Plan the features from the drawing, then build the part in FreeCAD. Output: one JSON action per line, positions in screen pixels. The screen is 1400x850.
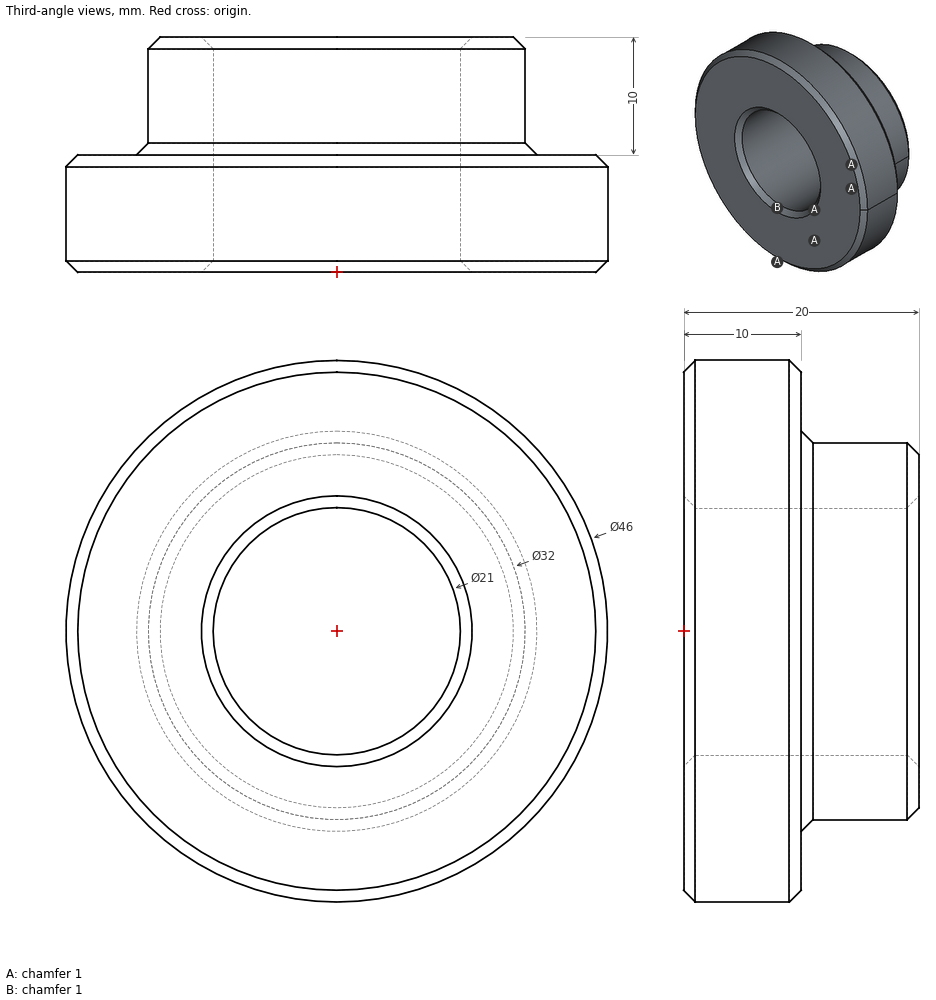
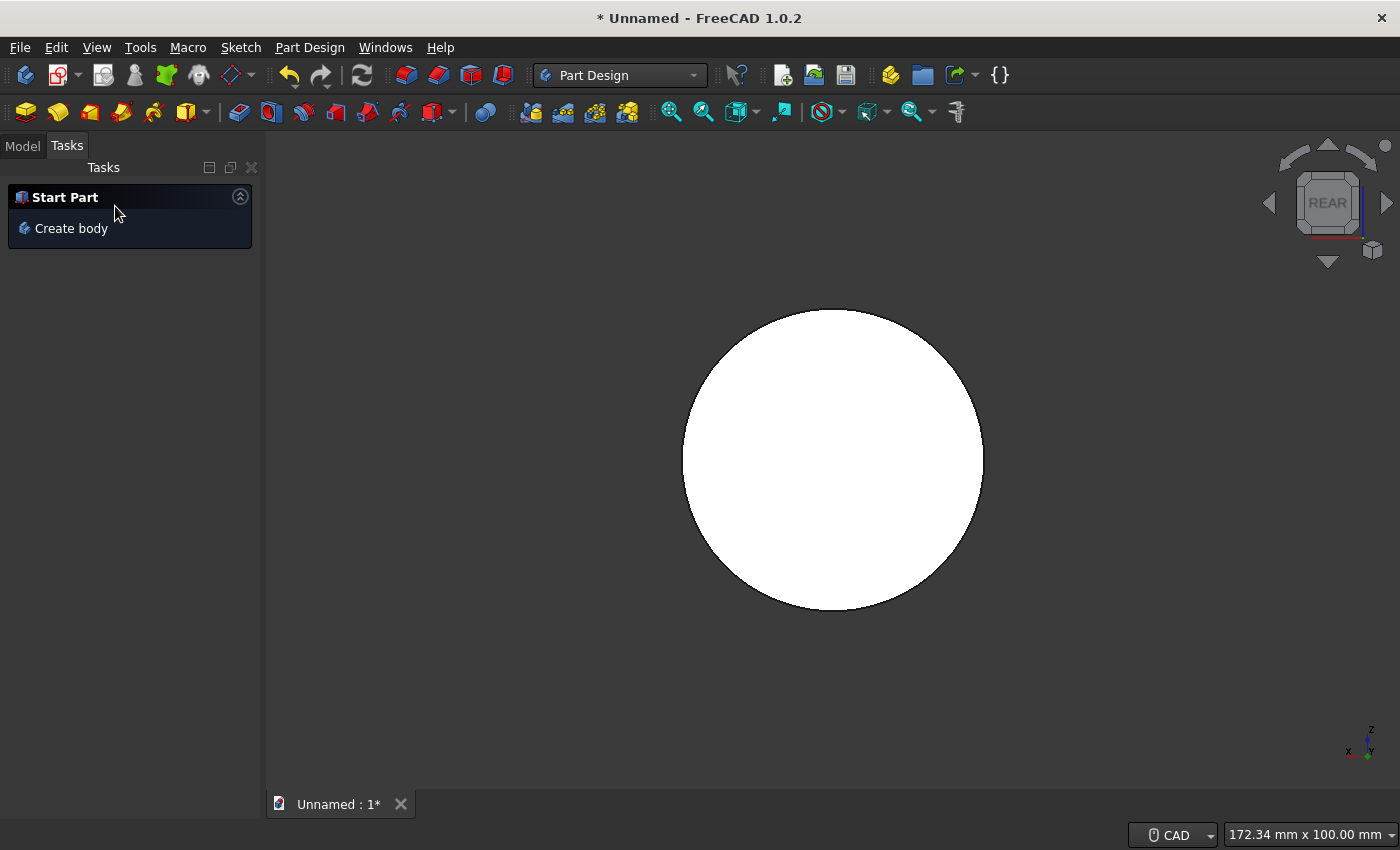
{"action": "left_click", "coordinate": [833, 459]}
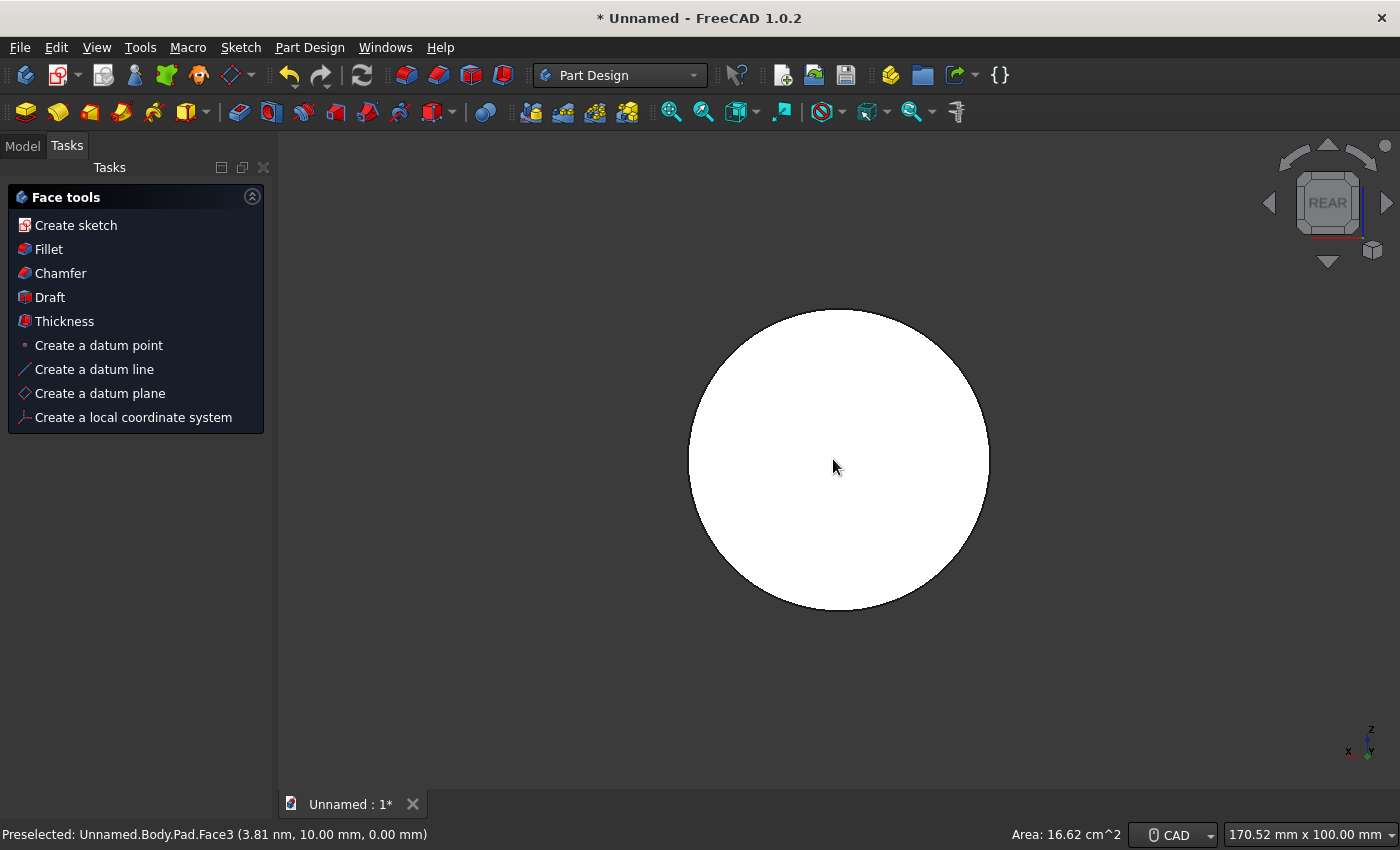
{"action": "left_click", "coordinate": [58, 76]}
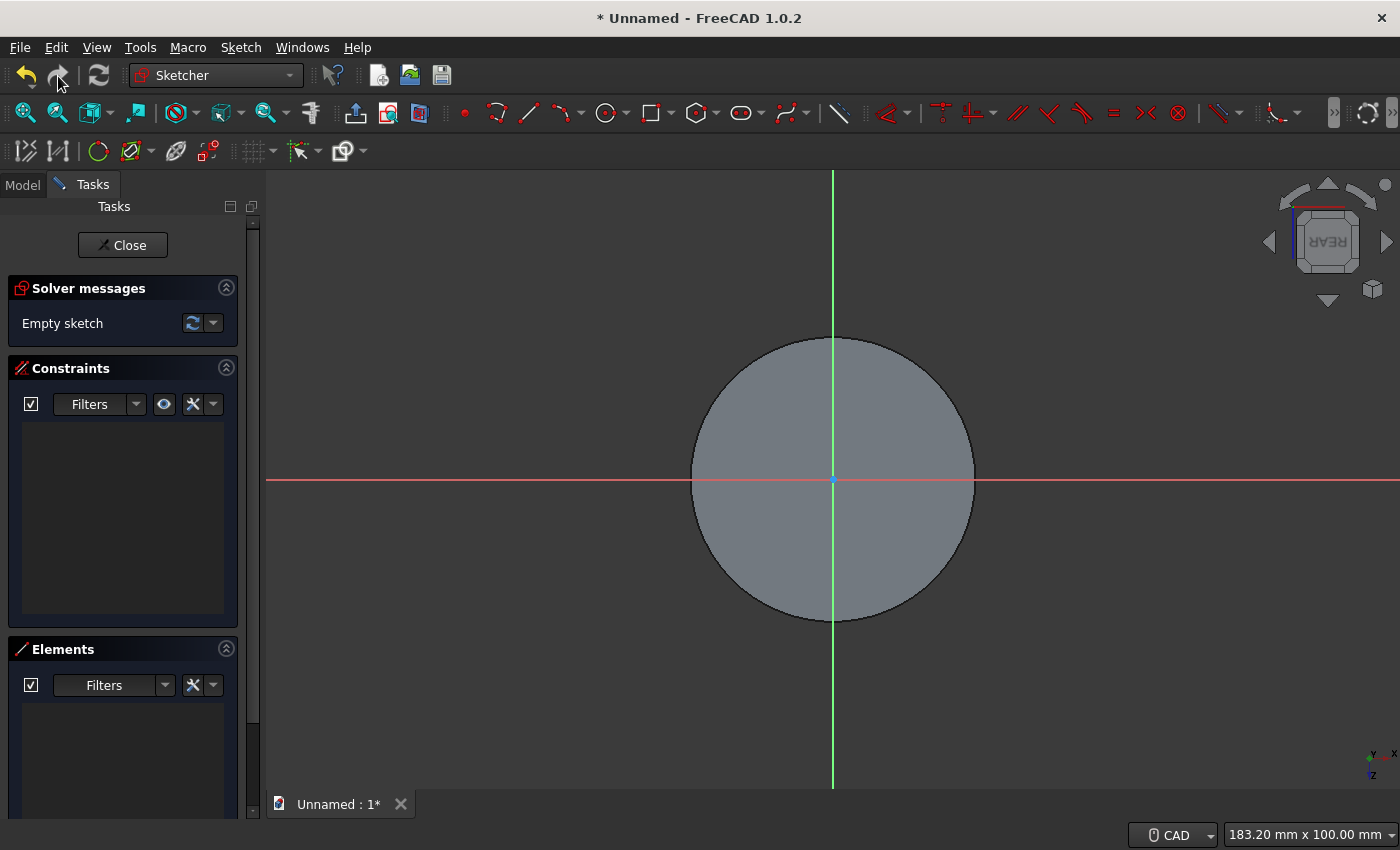
{"action": "scroll", "coordinate": [916, 480], "scroll_direction": "up", "scroll_amount": 3}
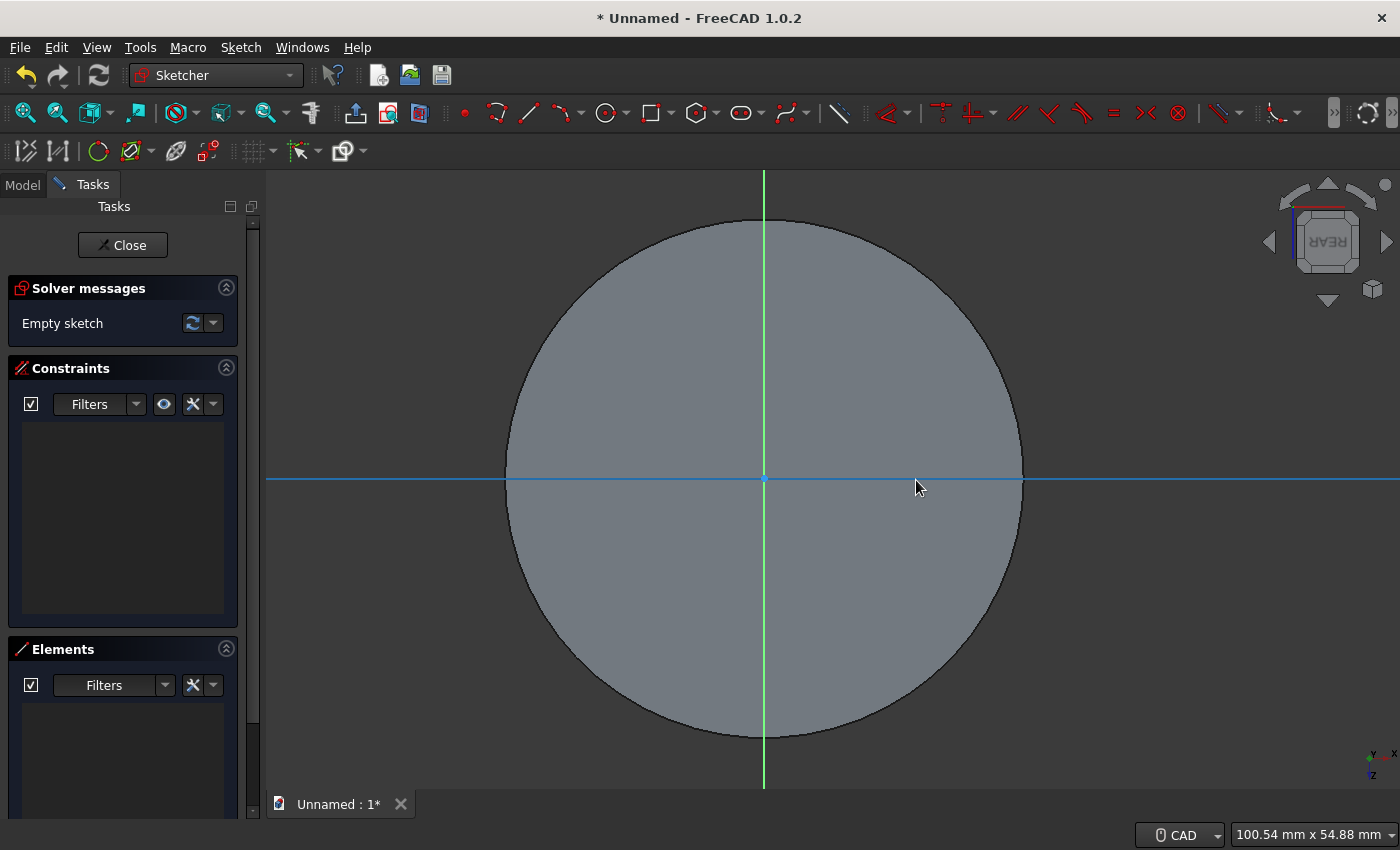
{"action": "key", "text": "g c"}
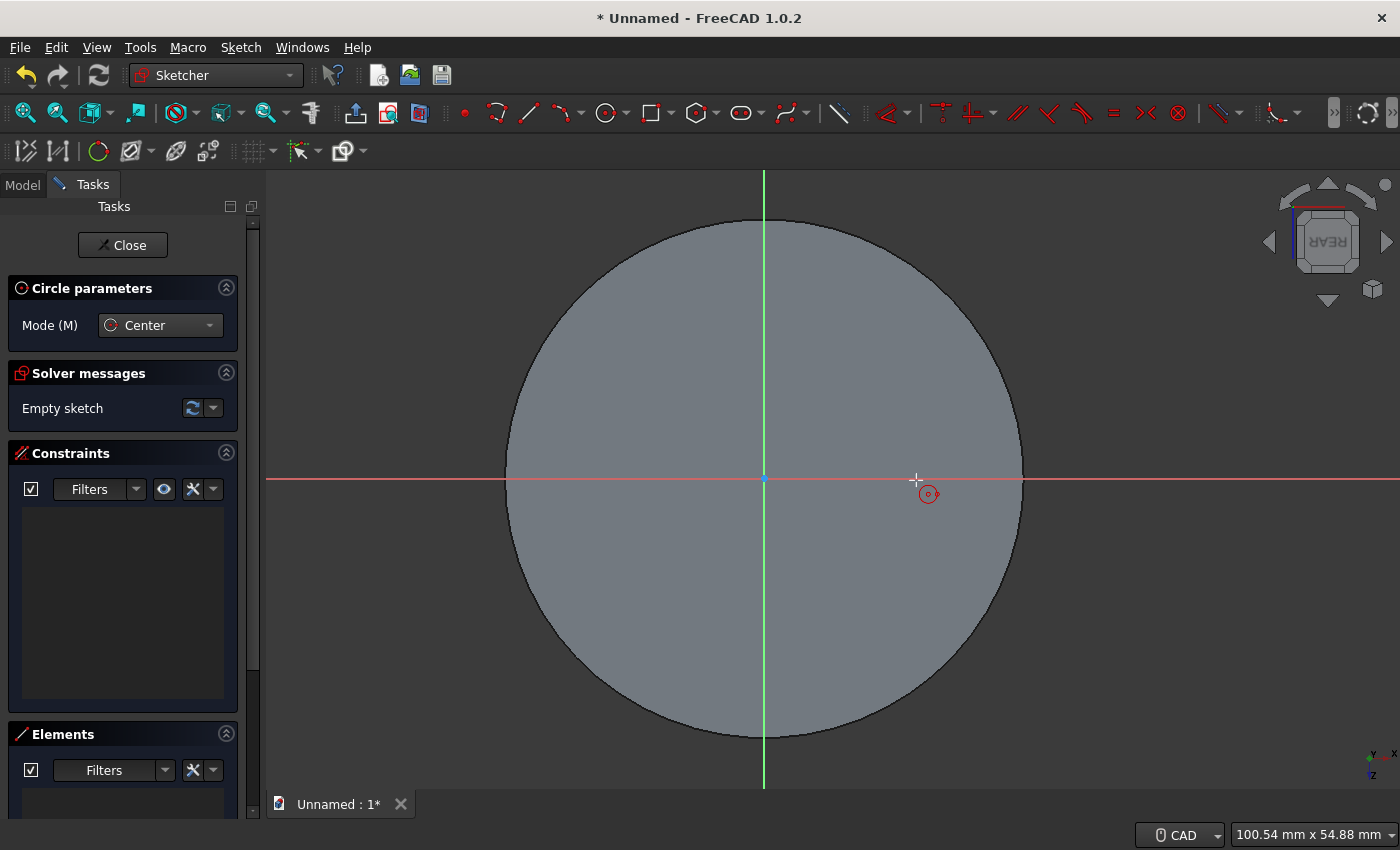
{"action": "left_click", "coordinate": [764, 479]}
{"action": "left_click", "coordinate": [892, 351]}
{"action": "key", "text": "Escape"}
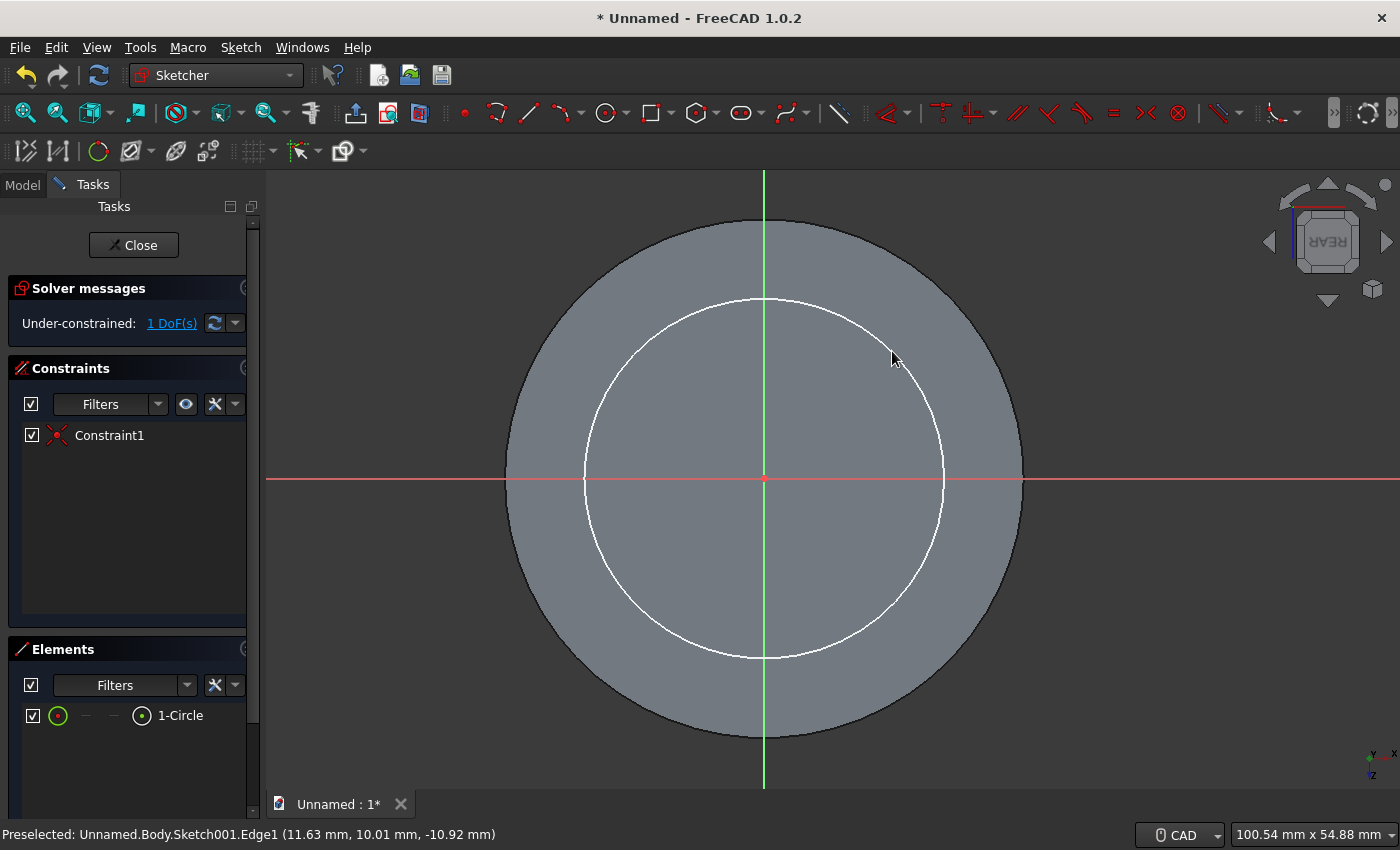
{"action": "left_click", "coordinate": [886, 114]}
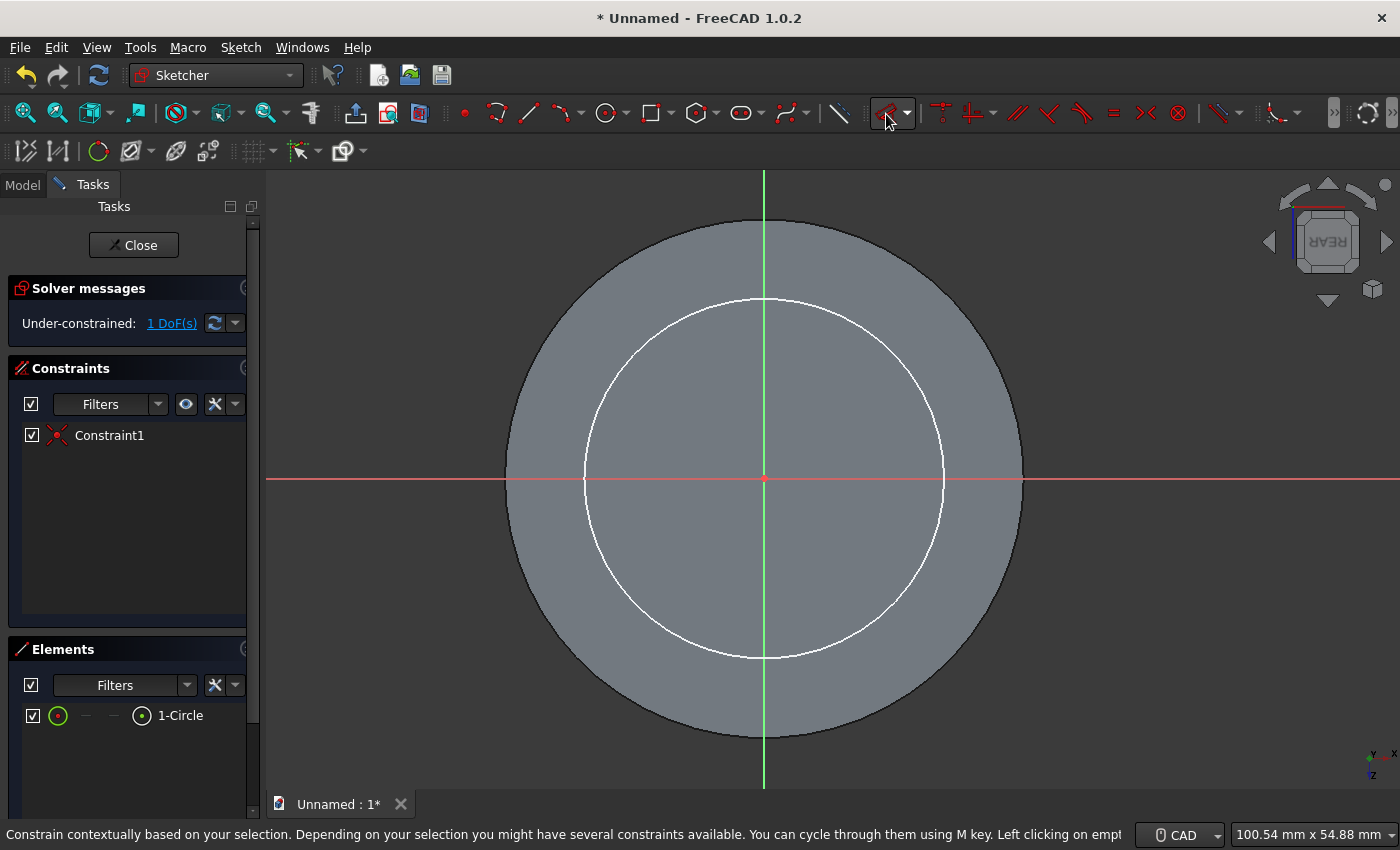
{"action": "left_click", "coordinate": [891, 351]}
{"action": "left_click", "coordinate": [914, 328]}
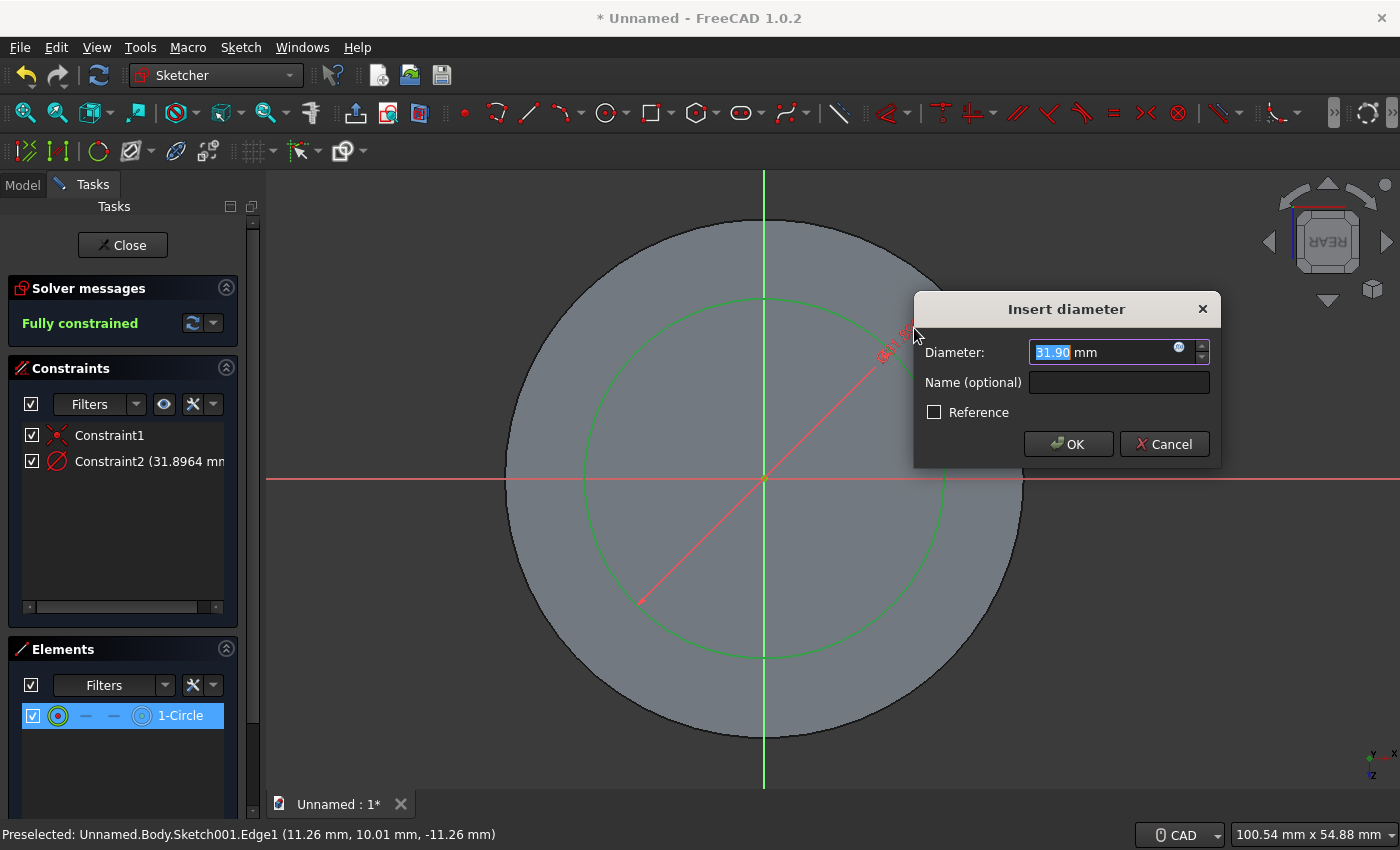
{"action": "type", "text": "32"}
{"action": "key", "text": "Return"}
{"action": "key", "text": "Escape"}